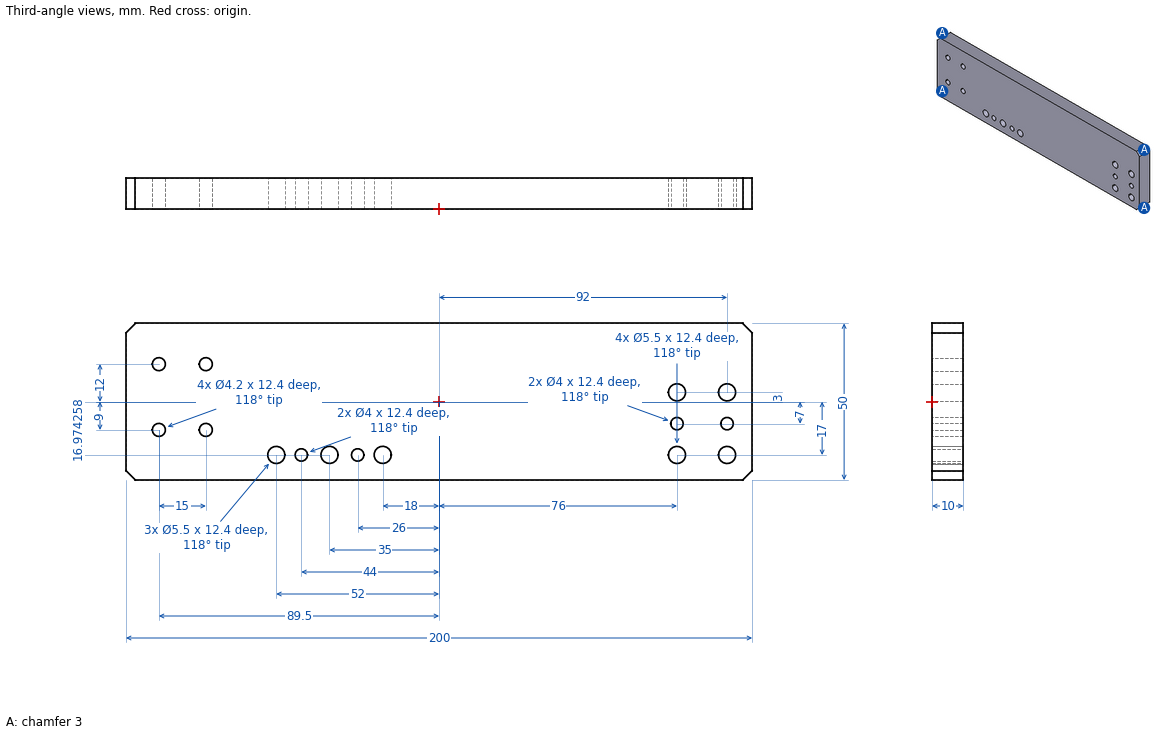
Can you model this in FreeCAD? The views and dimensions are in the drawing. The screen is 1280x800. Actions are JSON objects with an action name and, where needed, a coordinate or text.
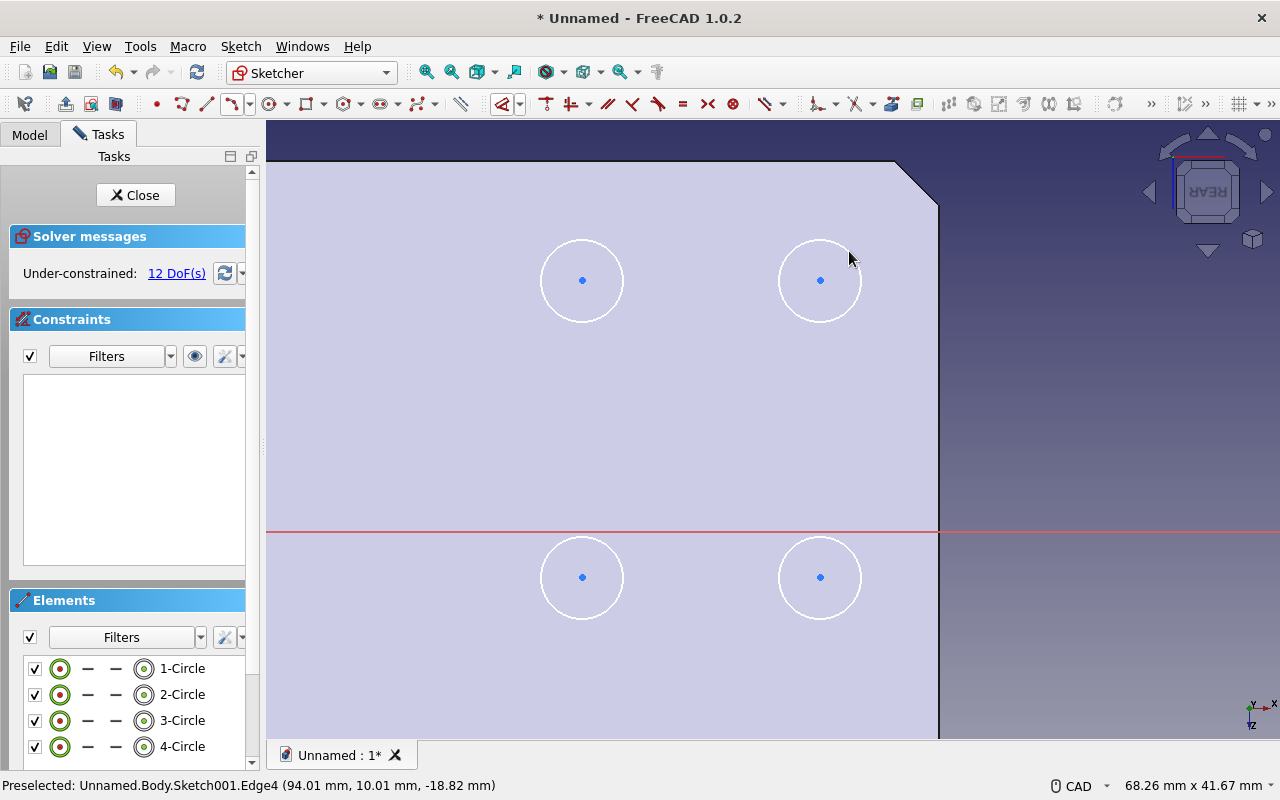
{"action": "left_click", "coordinate": [611, 252]}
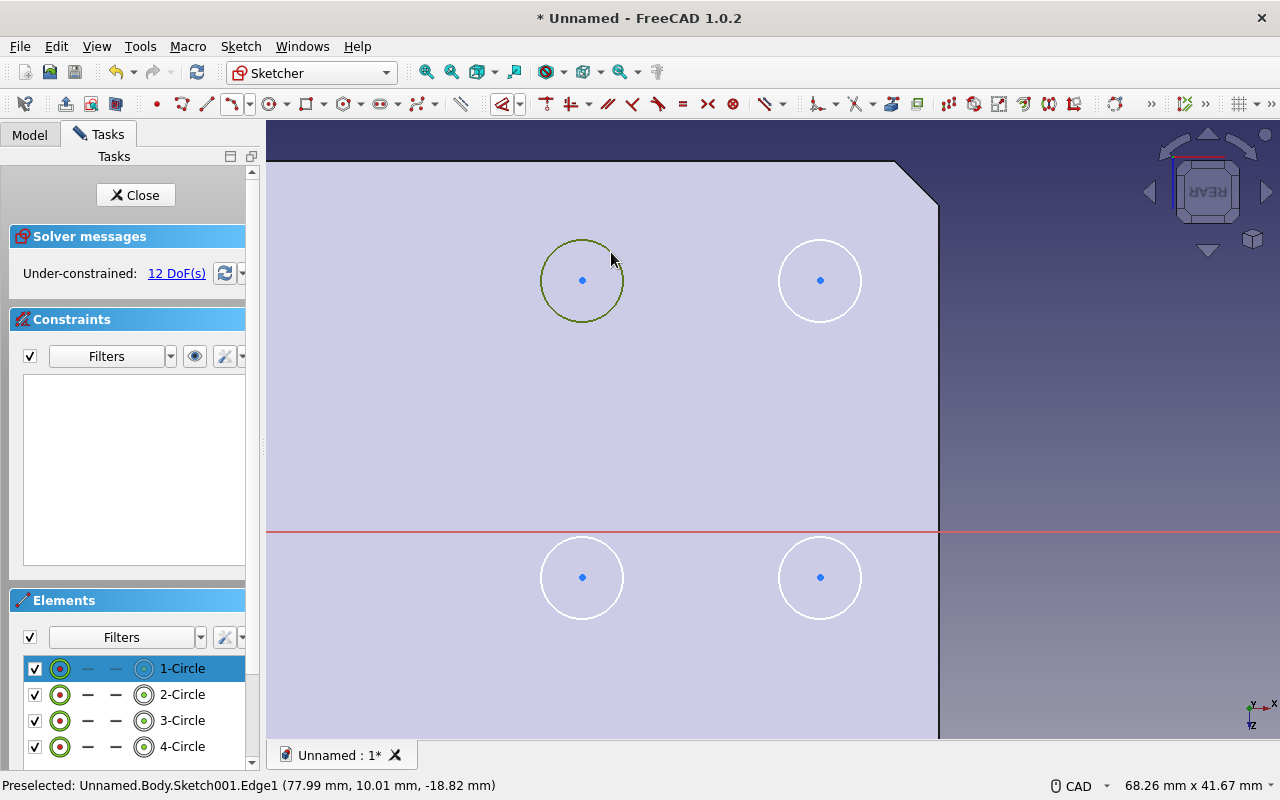
{"action": "left_click", "coordinate": [611, 549]}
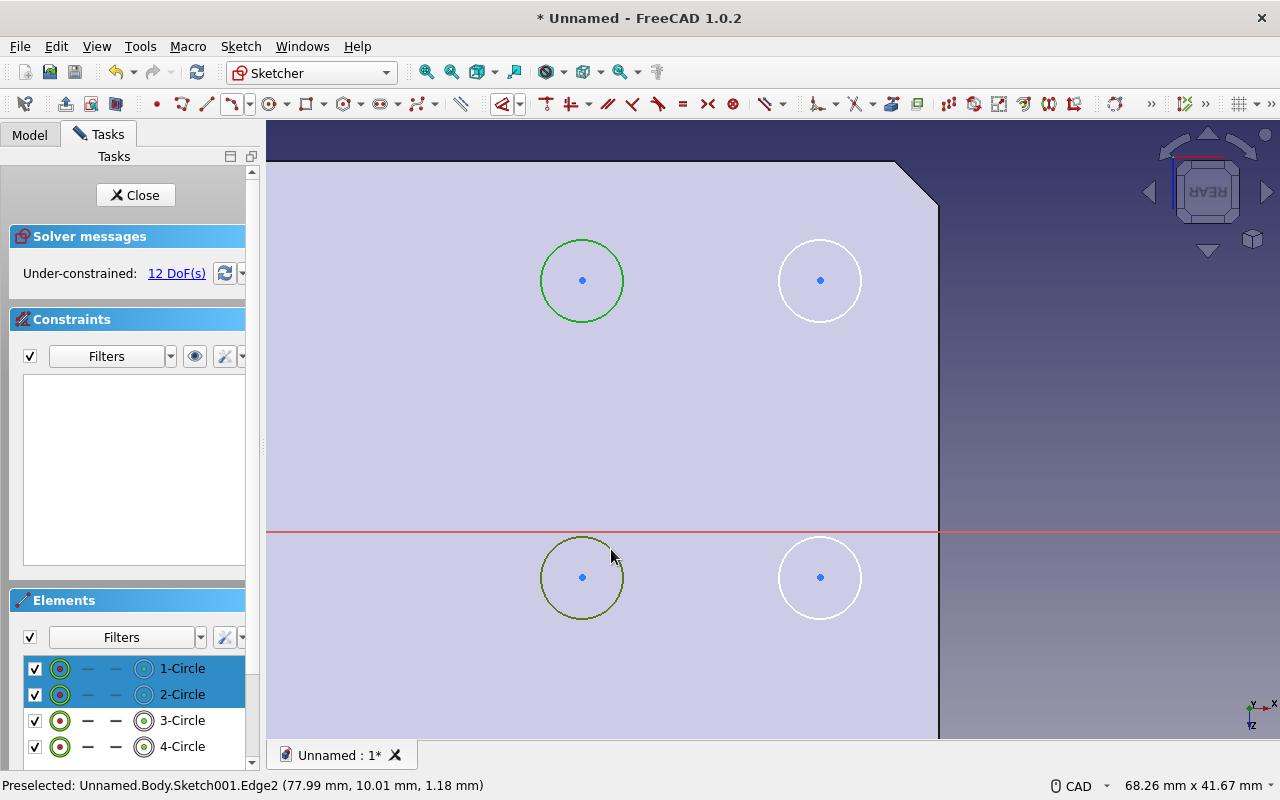
{"action": "left_click", "coordinate": [849, 549]}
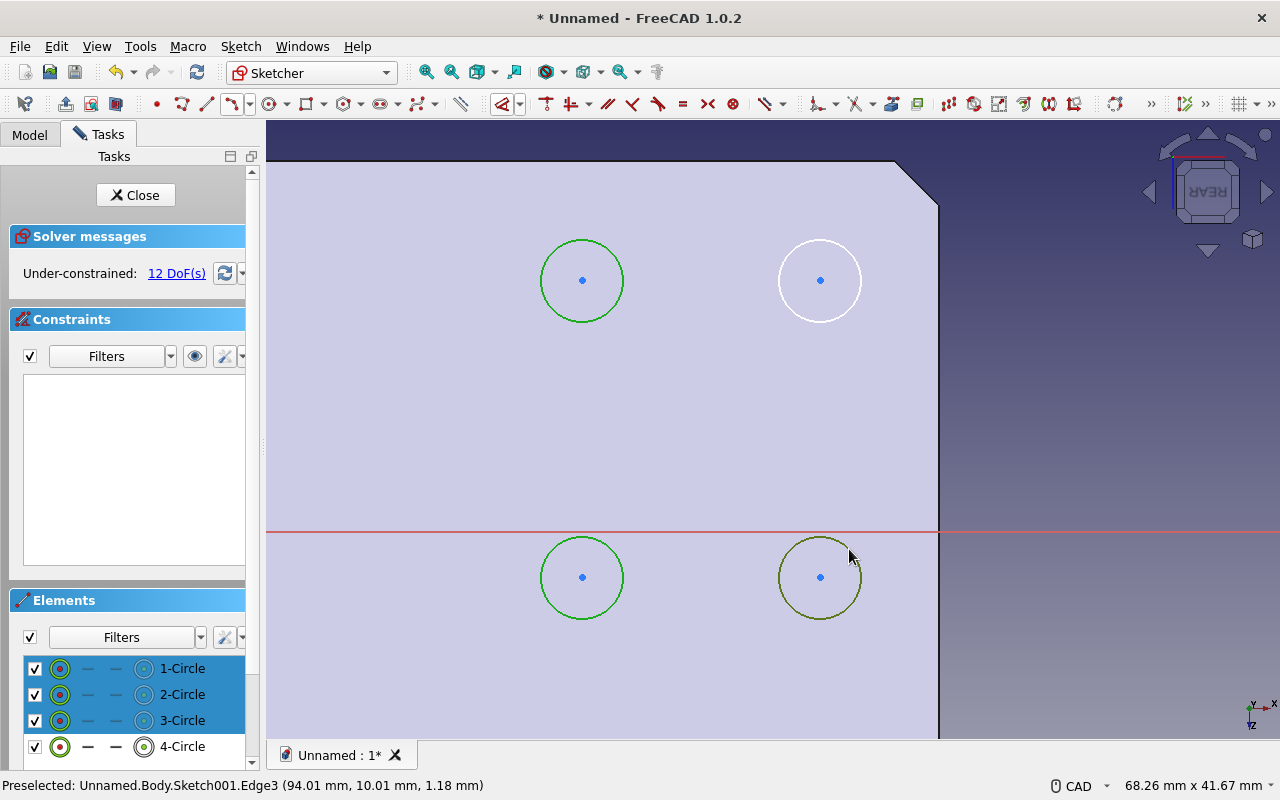
{"action": "left_click", "coordinate": [849, 252]}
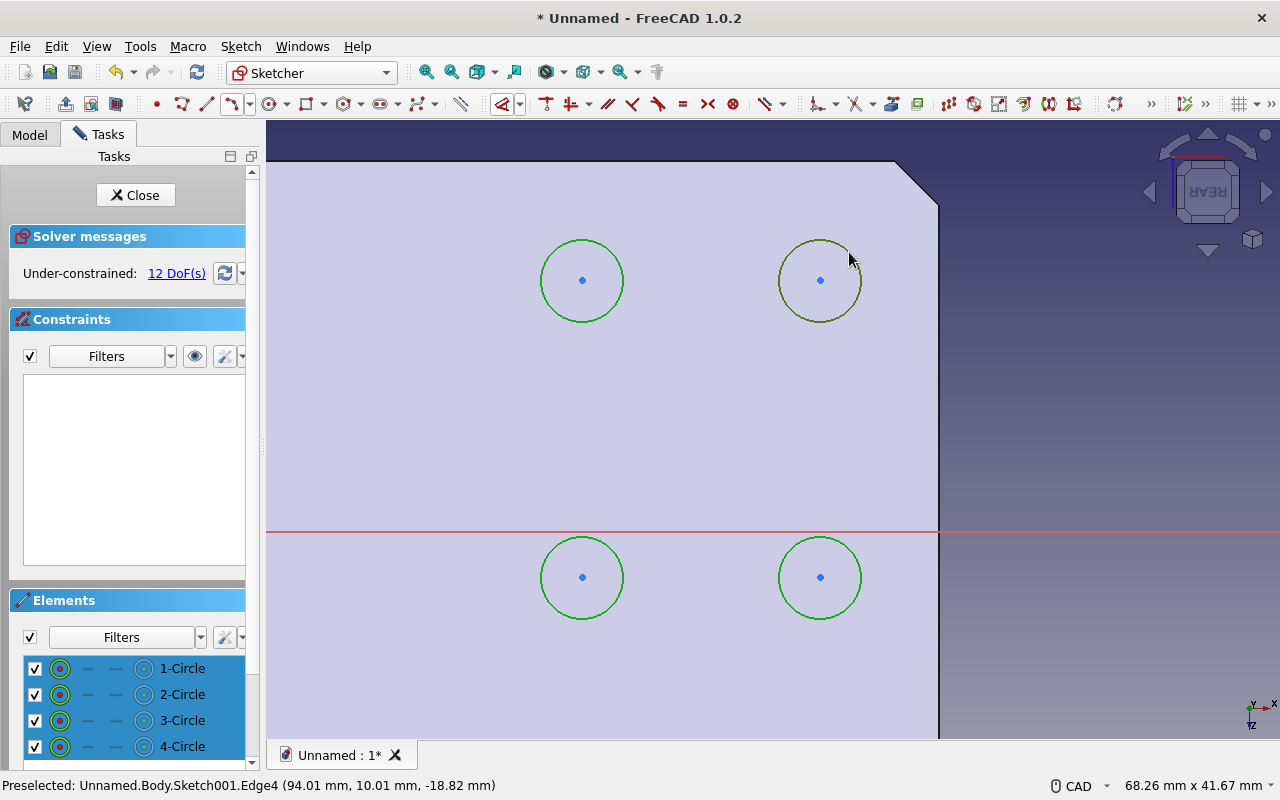
{"action": "left_click", "coordinate": [683, 104]}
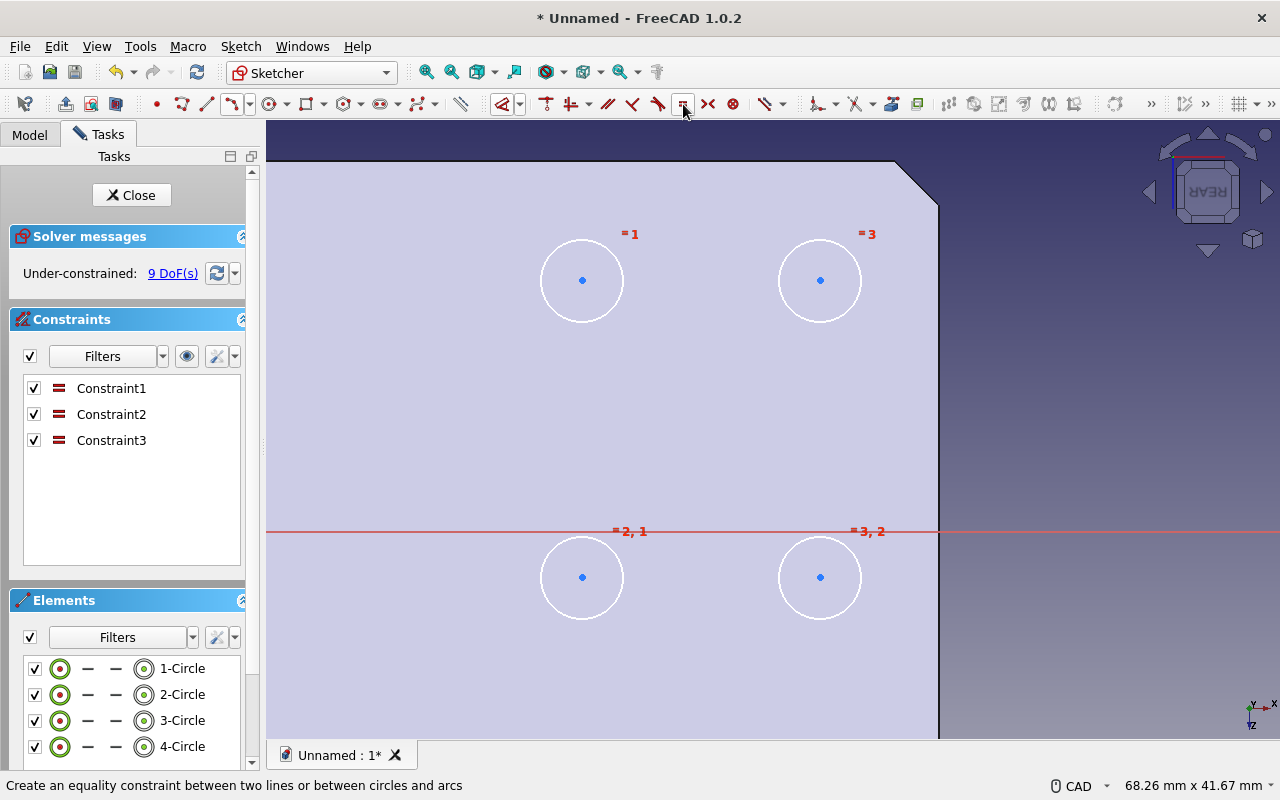
{"action": "left_click", "coordinate": [582, 281]}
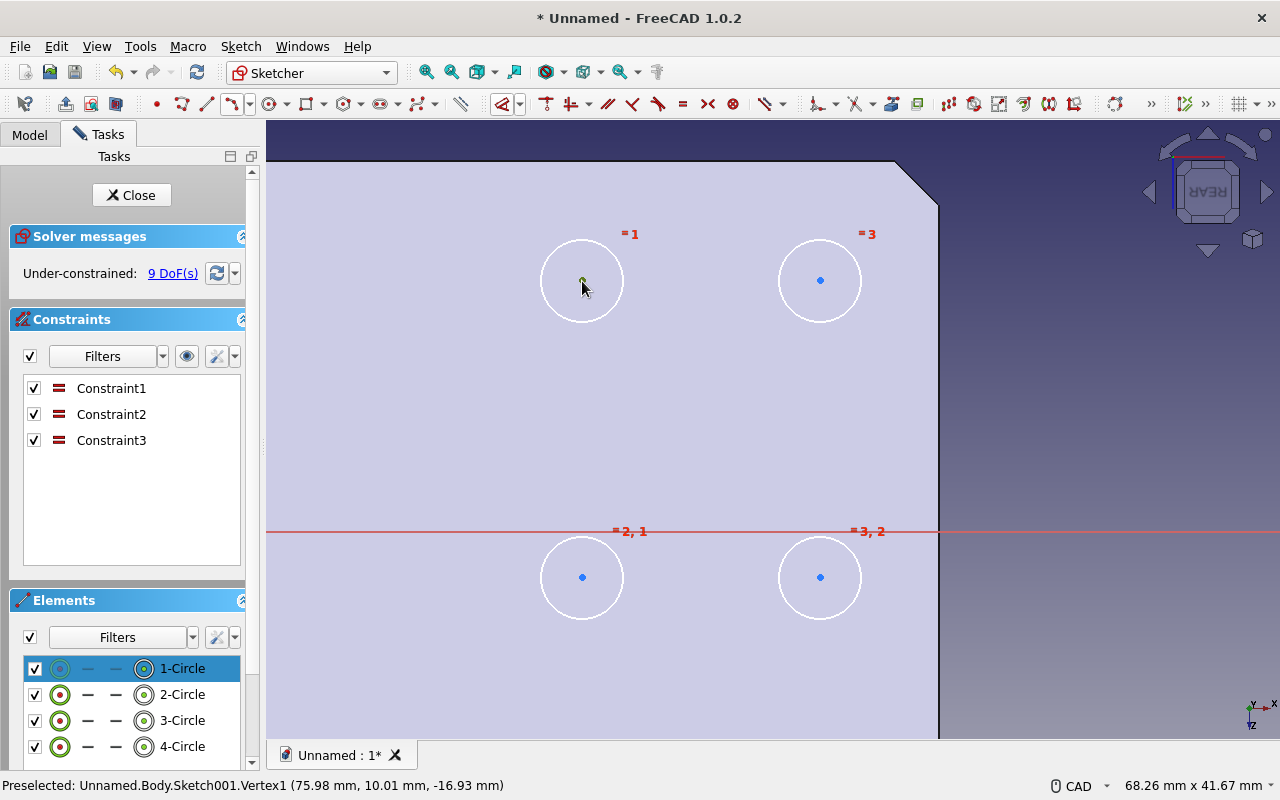
{"action": "left_click", "coordinate": [582, 578]}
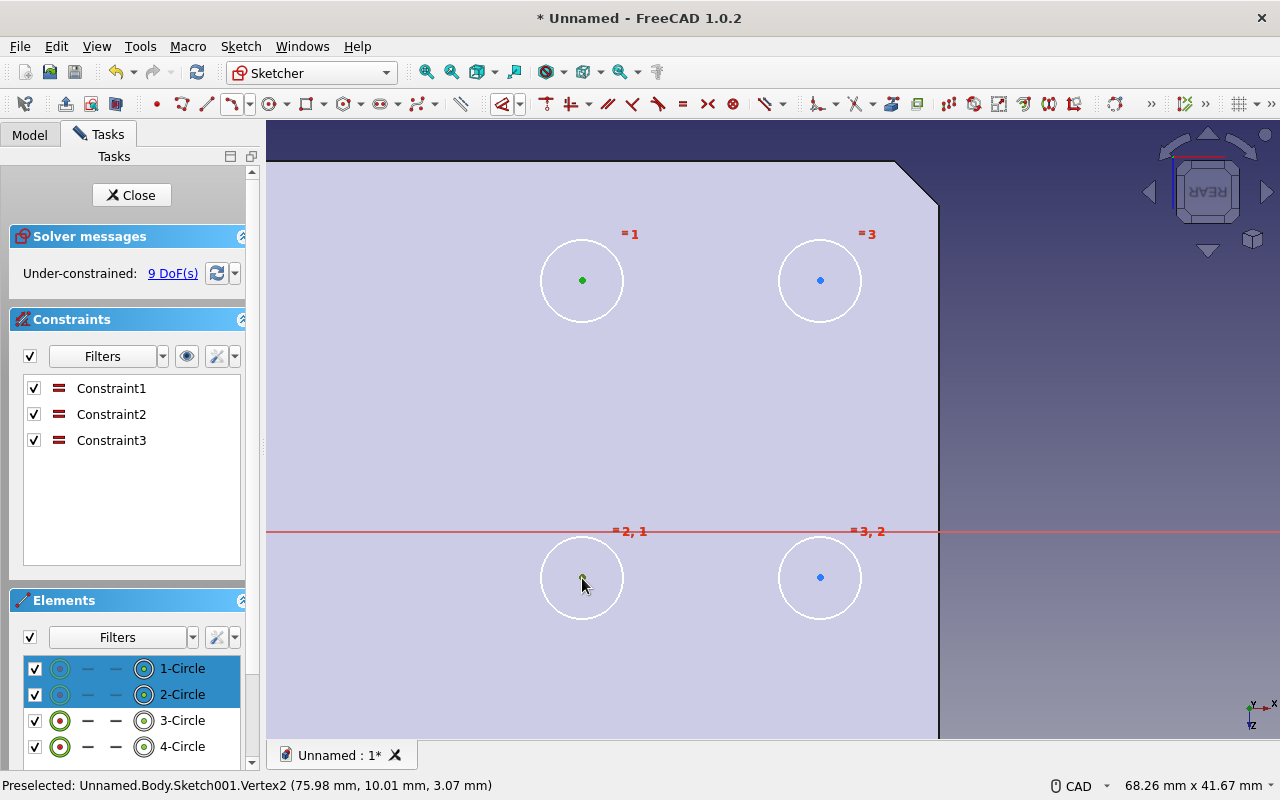
{"action": "key", "text": "v"}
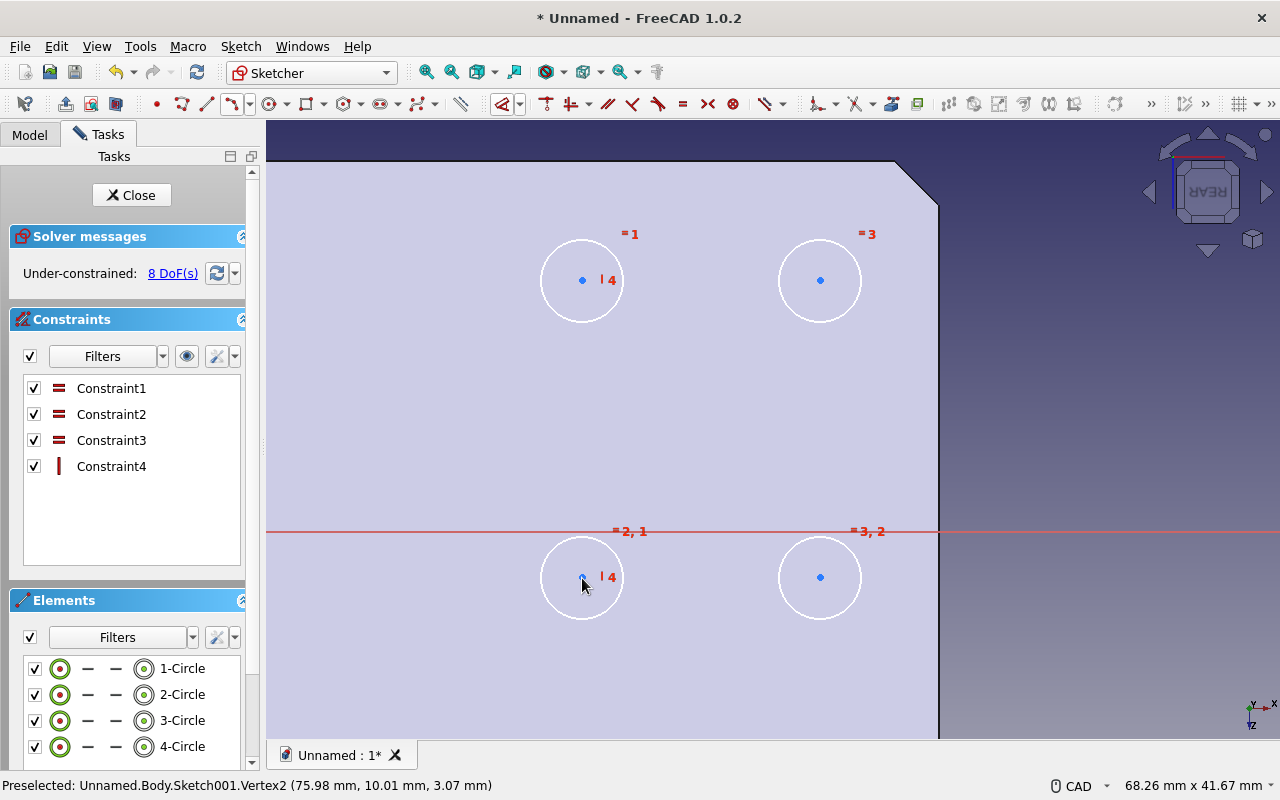
{"action": "left_click", "coordinate": [582, 578]}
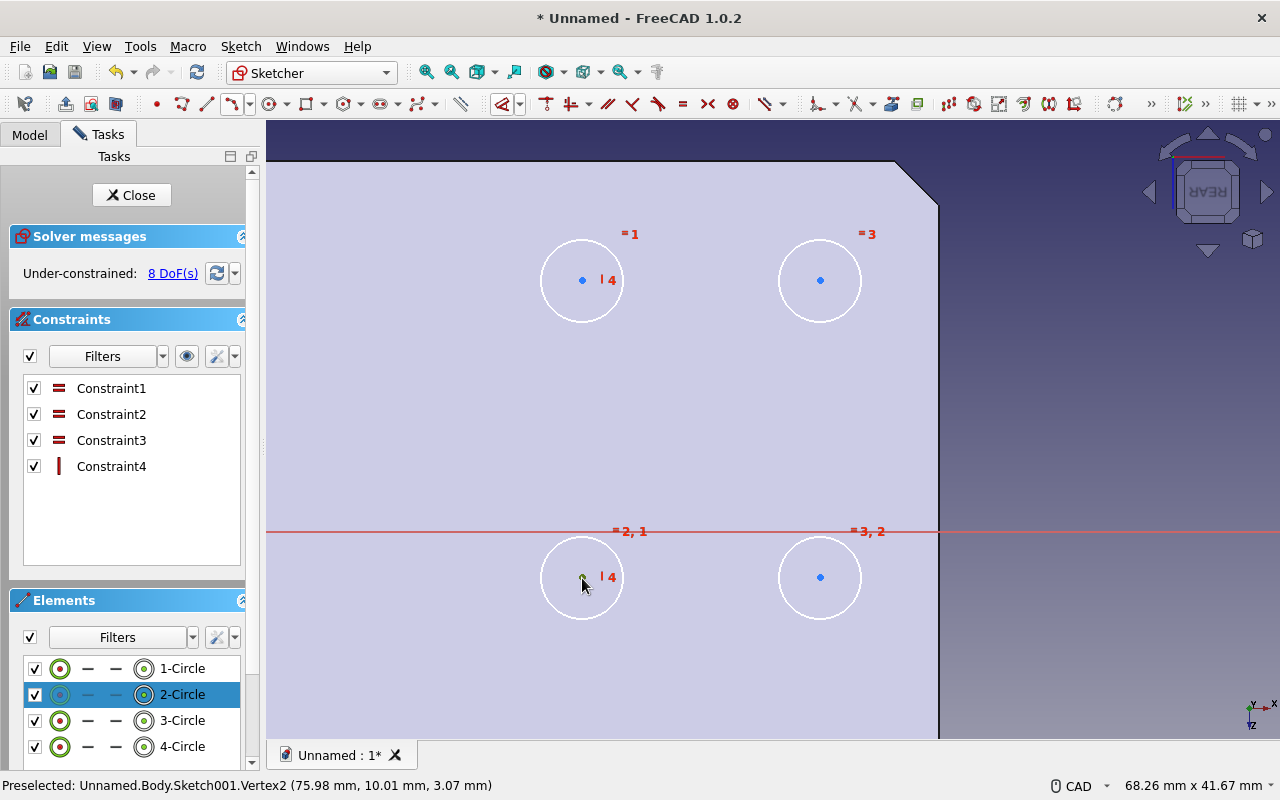
{"action": "left_click", "coordinate": [820, 578]}